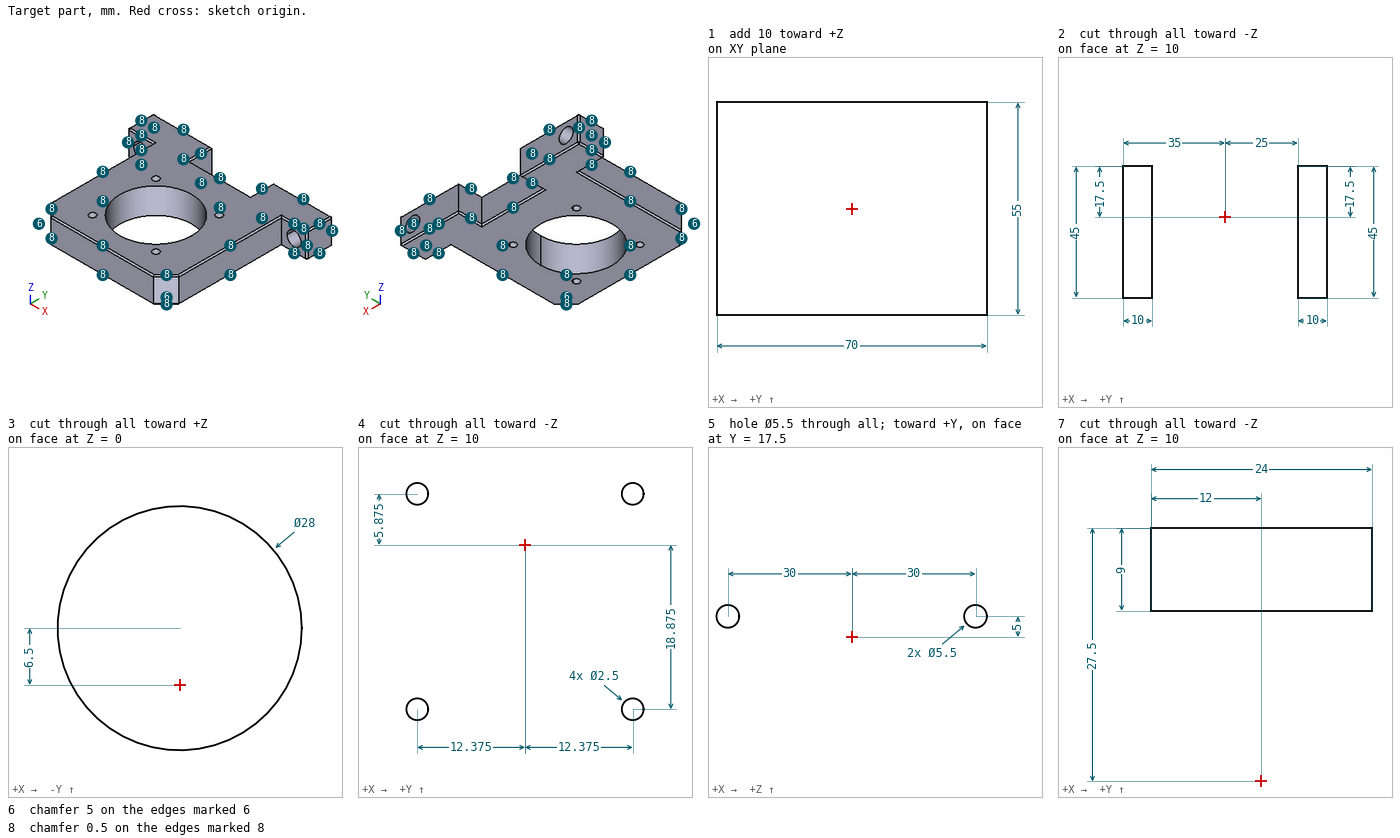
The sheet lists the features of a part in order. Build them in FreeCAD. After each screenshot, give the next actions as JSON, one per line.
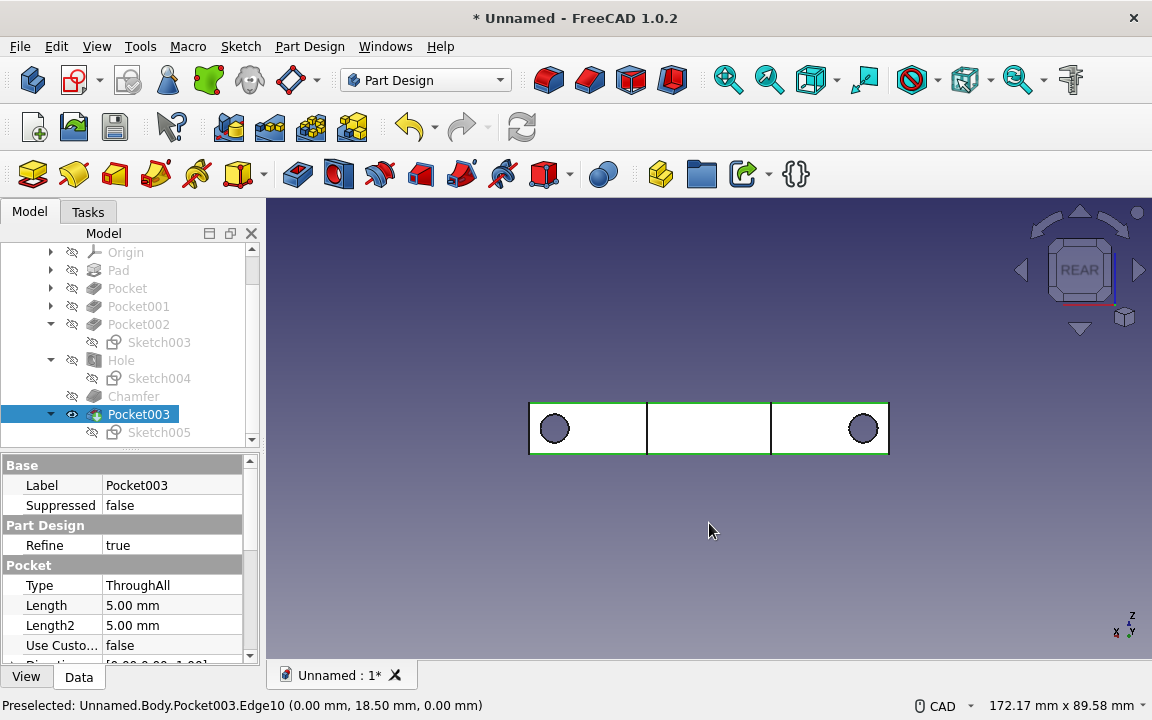
{"action": "left_click", "coordinate": [729, 80]}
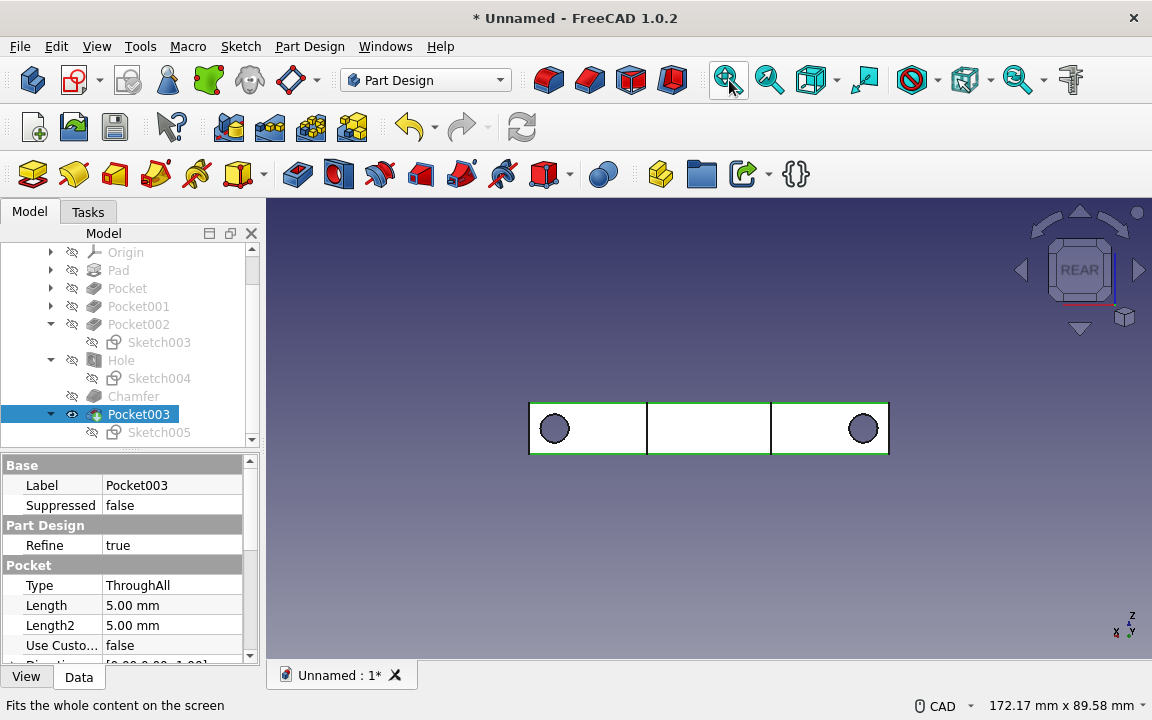
{"action": "key", "text": "6"}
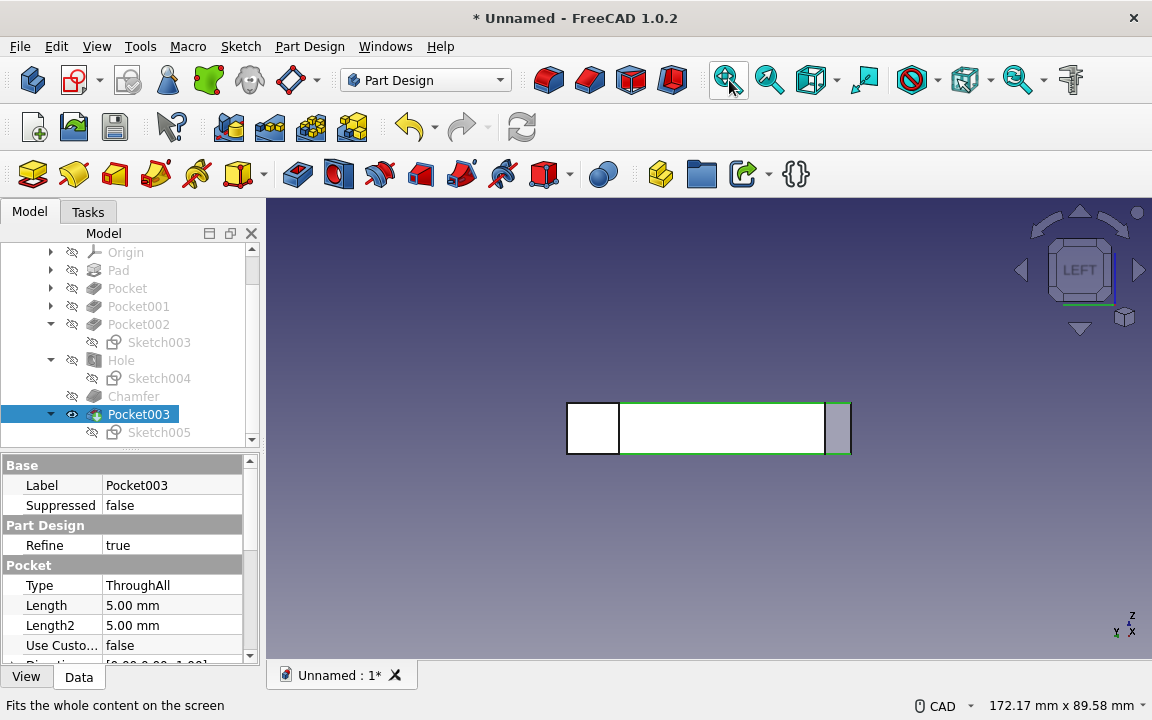
{"action": "left_click", "coordinate": [729, 80]}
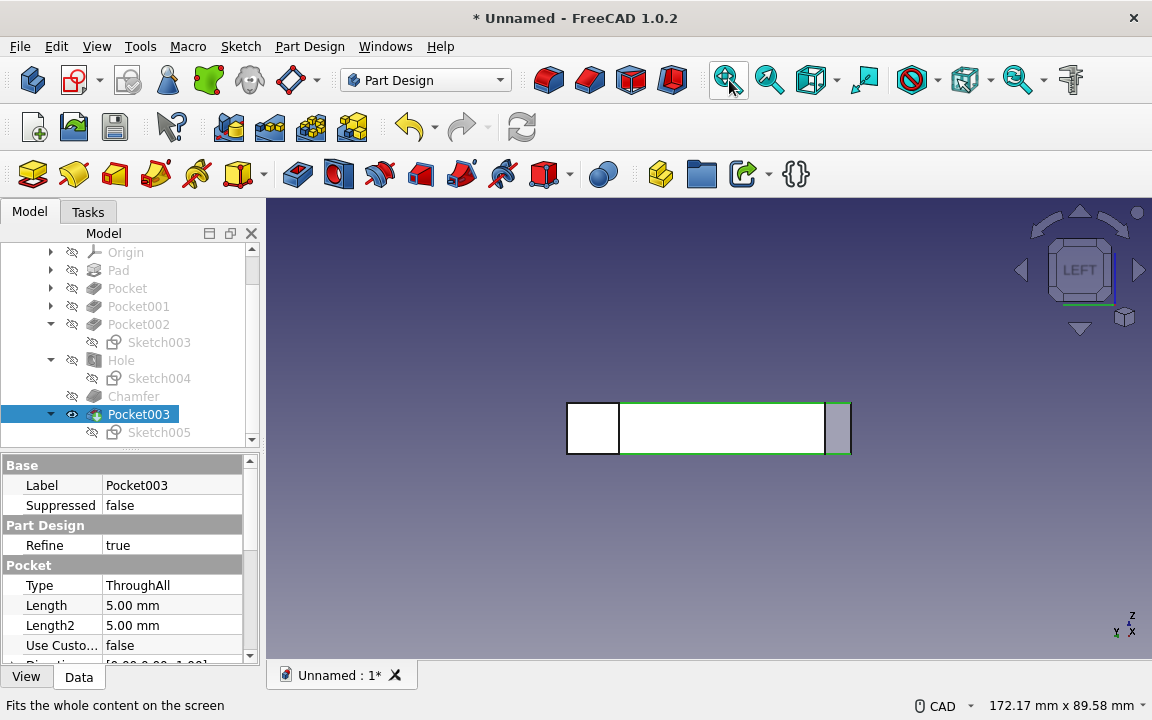
{"action": "left_click", "coordinate": [593, 427], "text": "ctrl"}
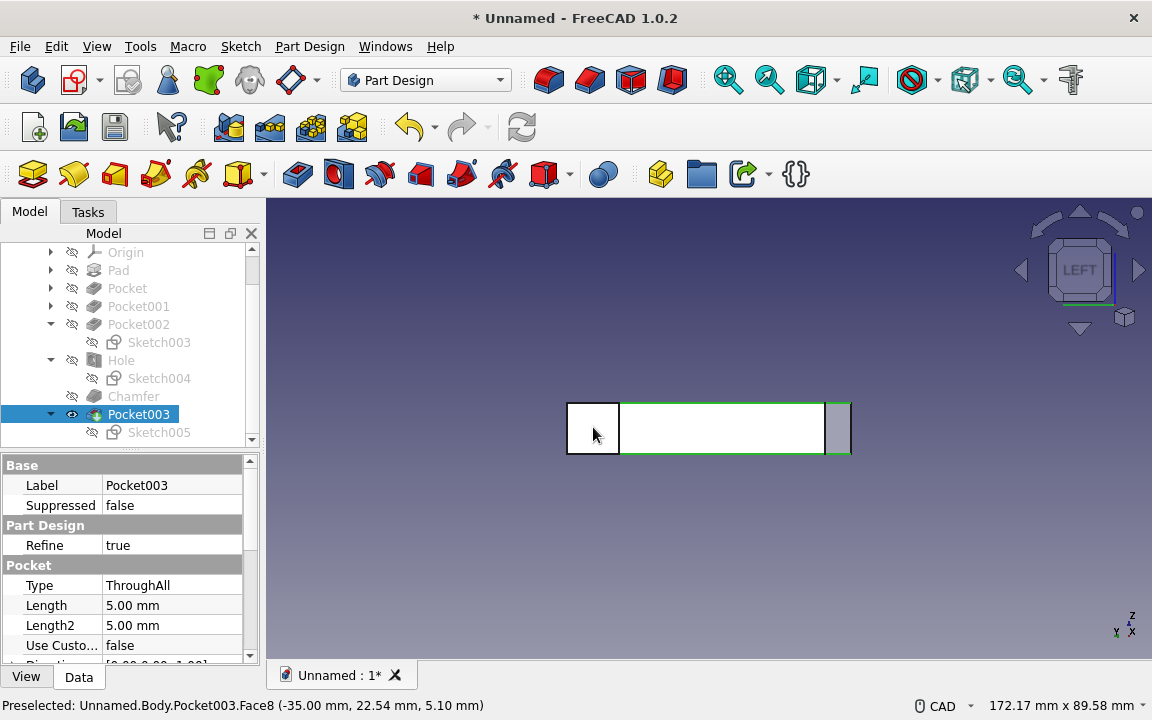
{"action": "left_click", "coordinate": [590, 80]}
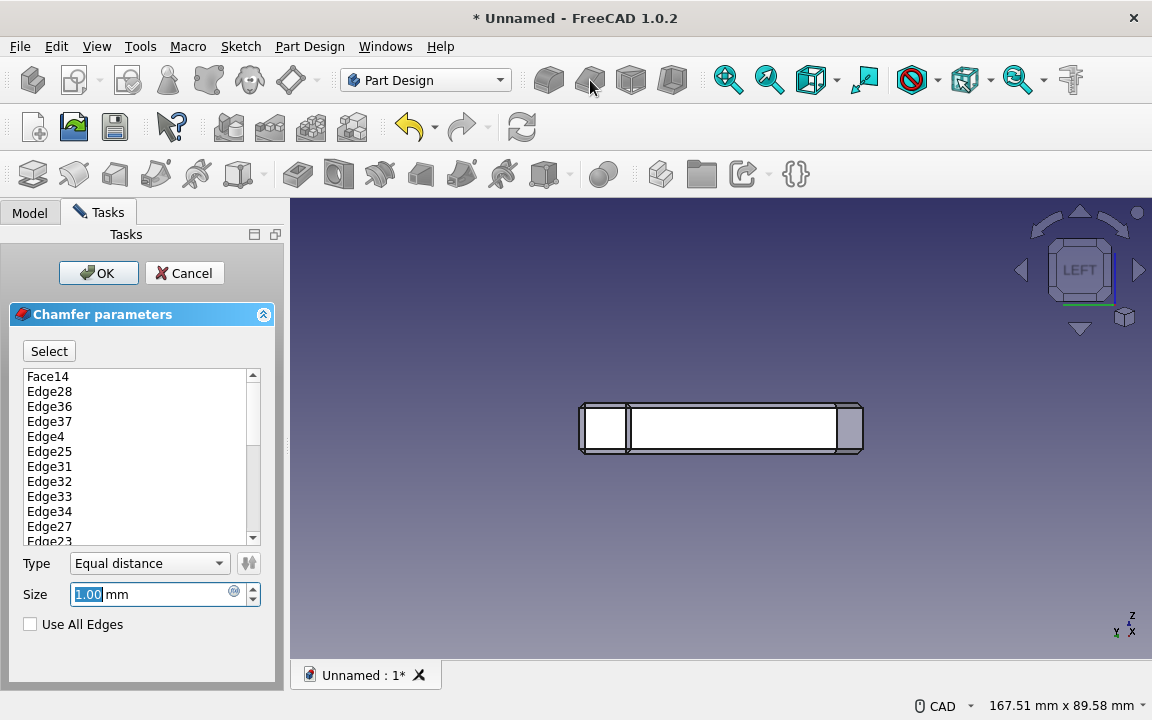
{"action": "type", "text": "0.5"}
{"action": "key", "text": "Tab"}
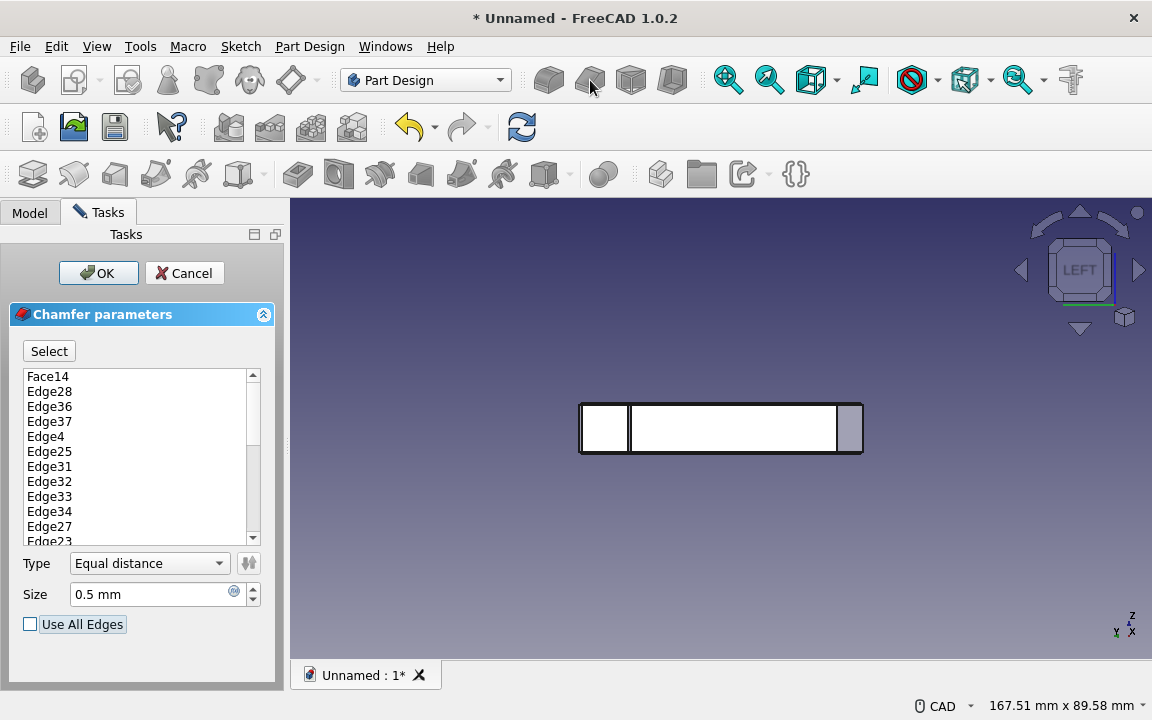
{"action": "left_click", "coordinate": [99, 273]}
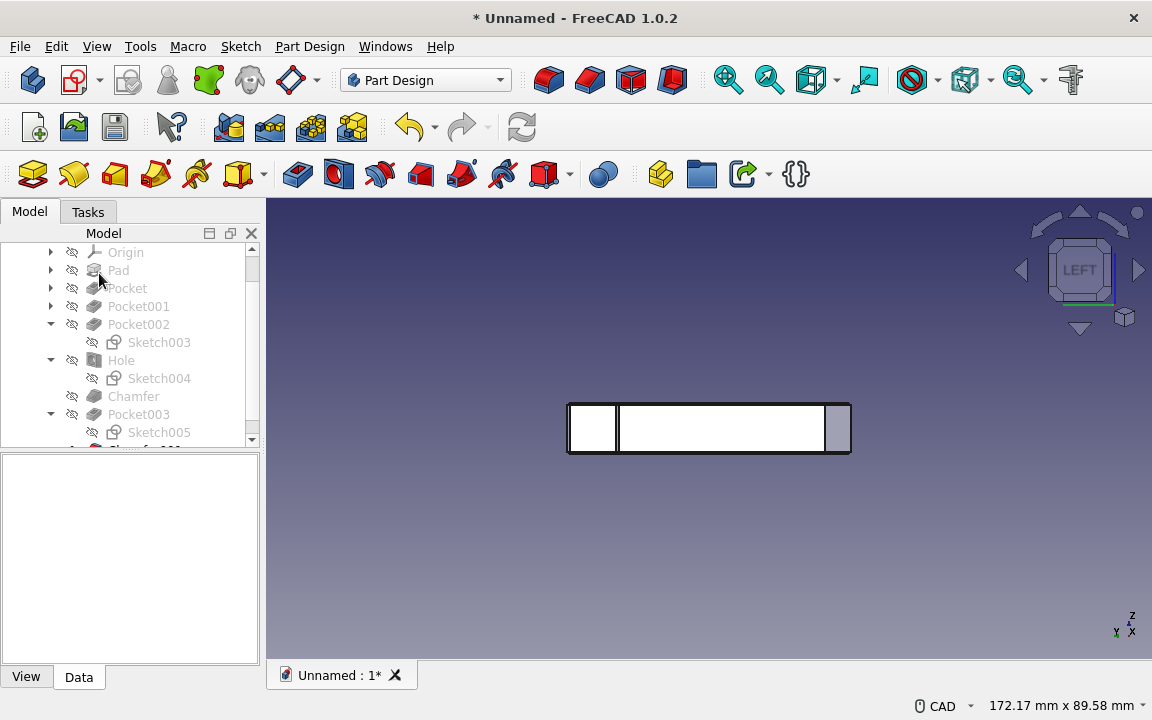
{"action": "key", "text": "0"}